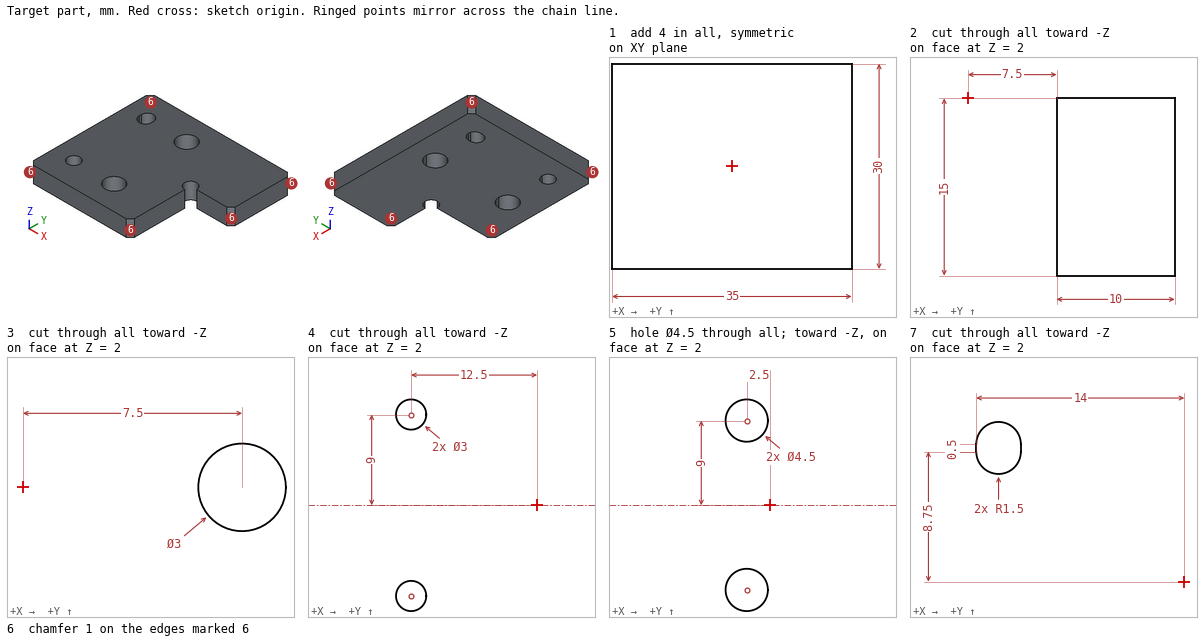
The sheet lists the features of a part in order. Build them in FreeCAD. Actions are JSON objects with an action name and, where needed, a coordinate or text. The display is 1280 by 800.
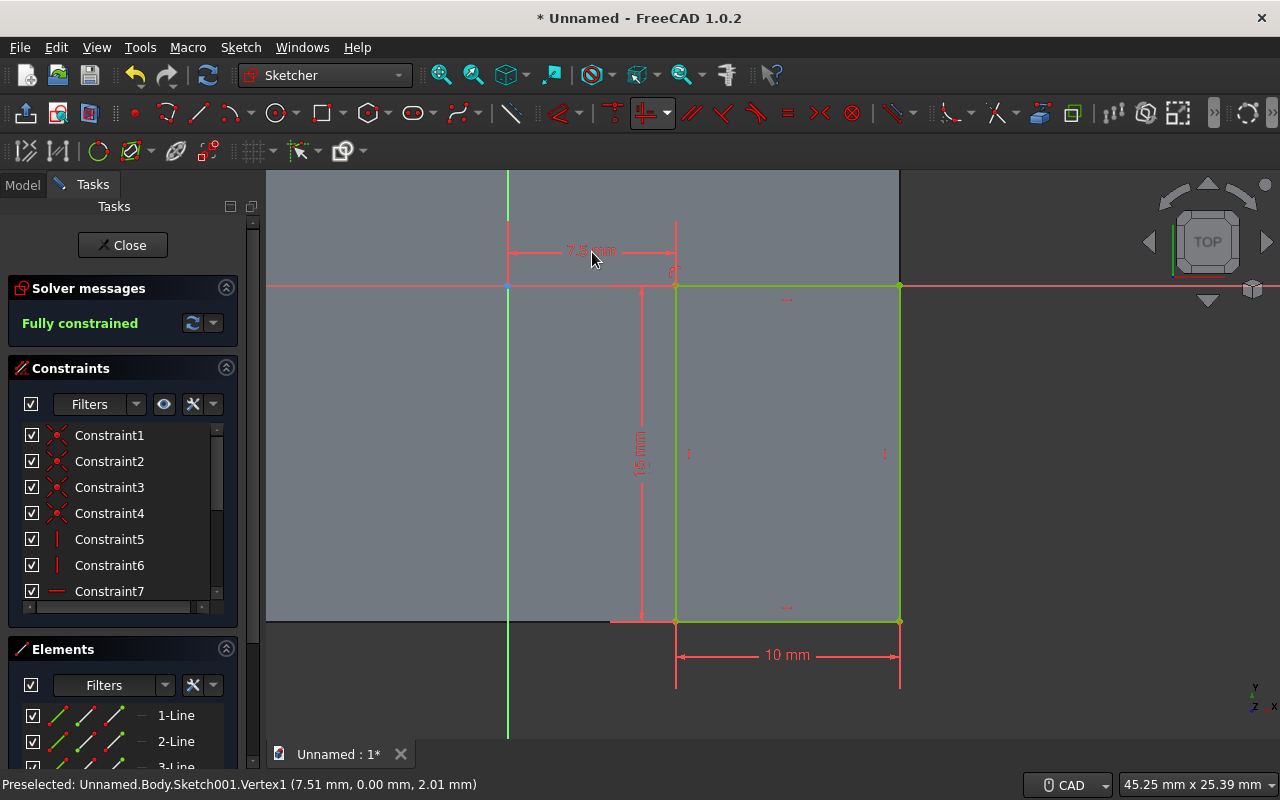
{"action": "left_click", "coordinate": [123, 245]}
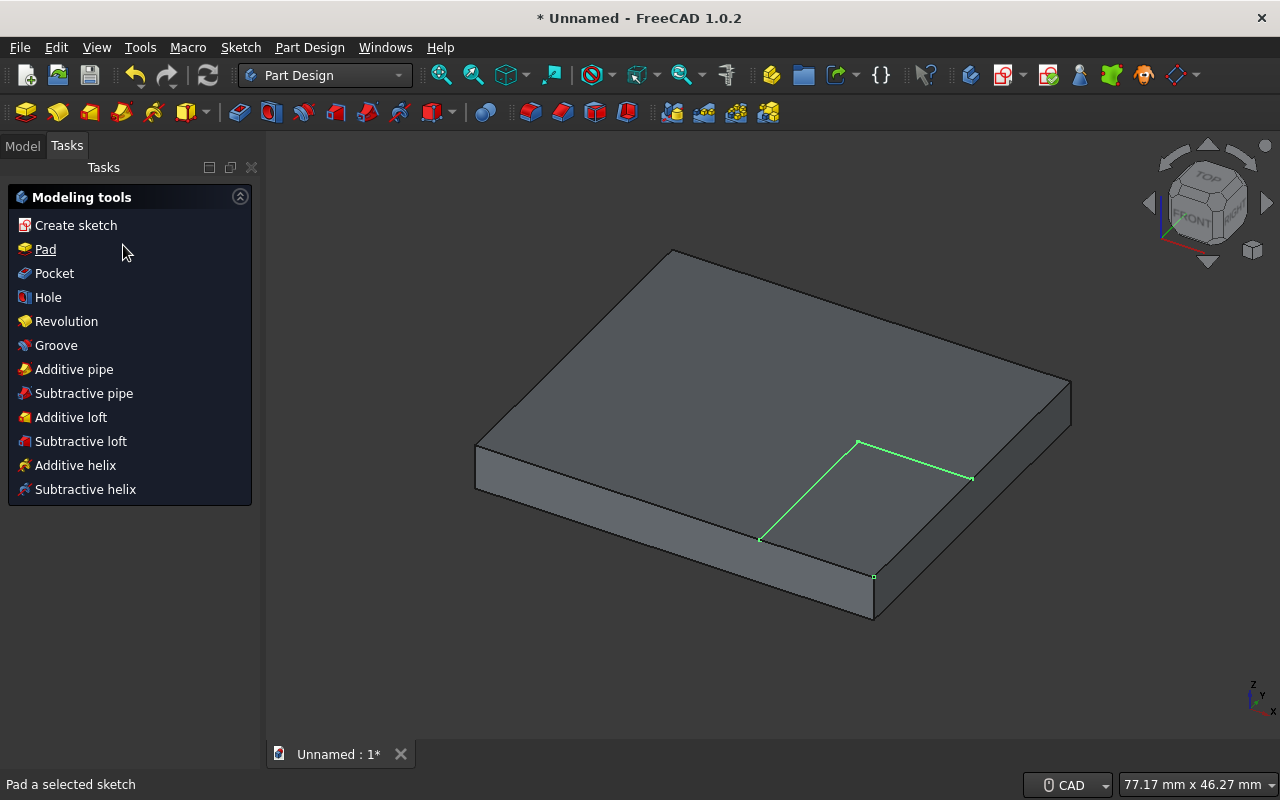
{"action": "left_click", "coordinate": [240, 112]}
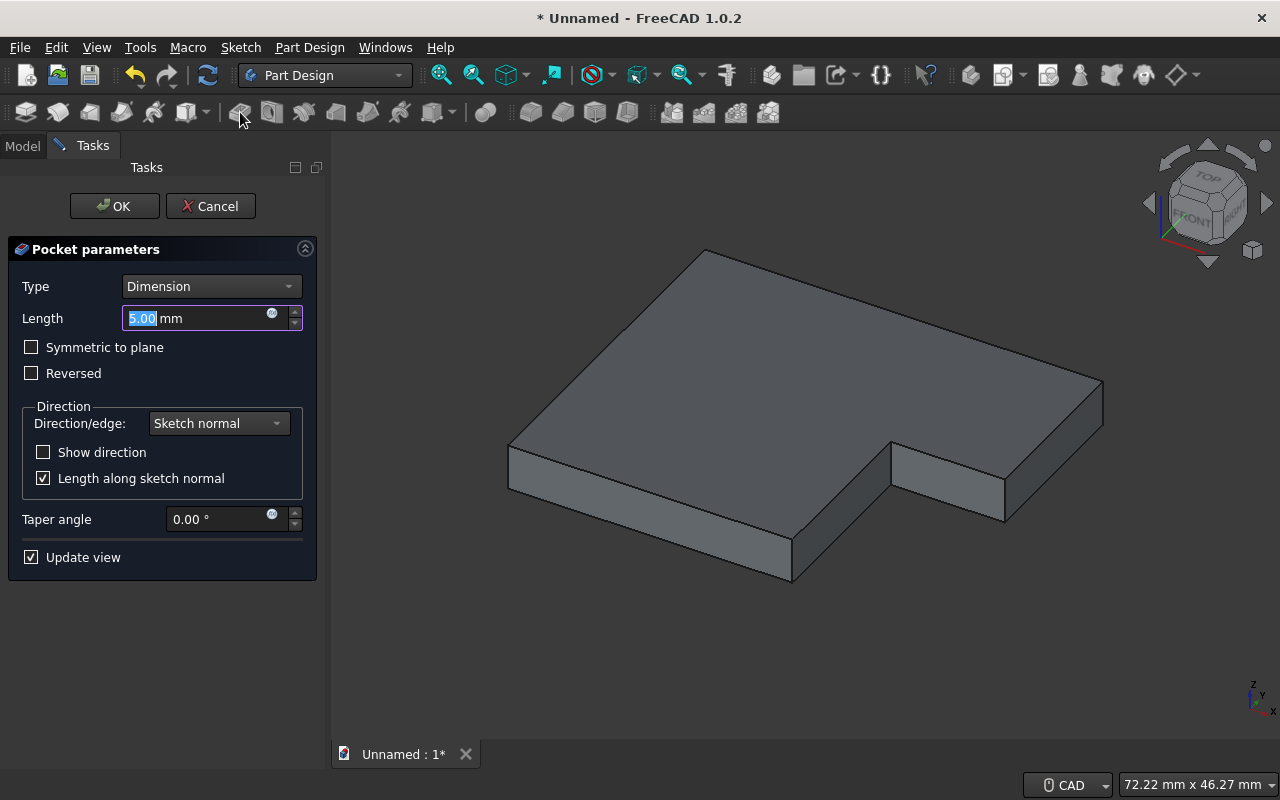
{"action": "left_click", "coordinate": [212, 286]}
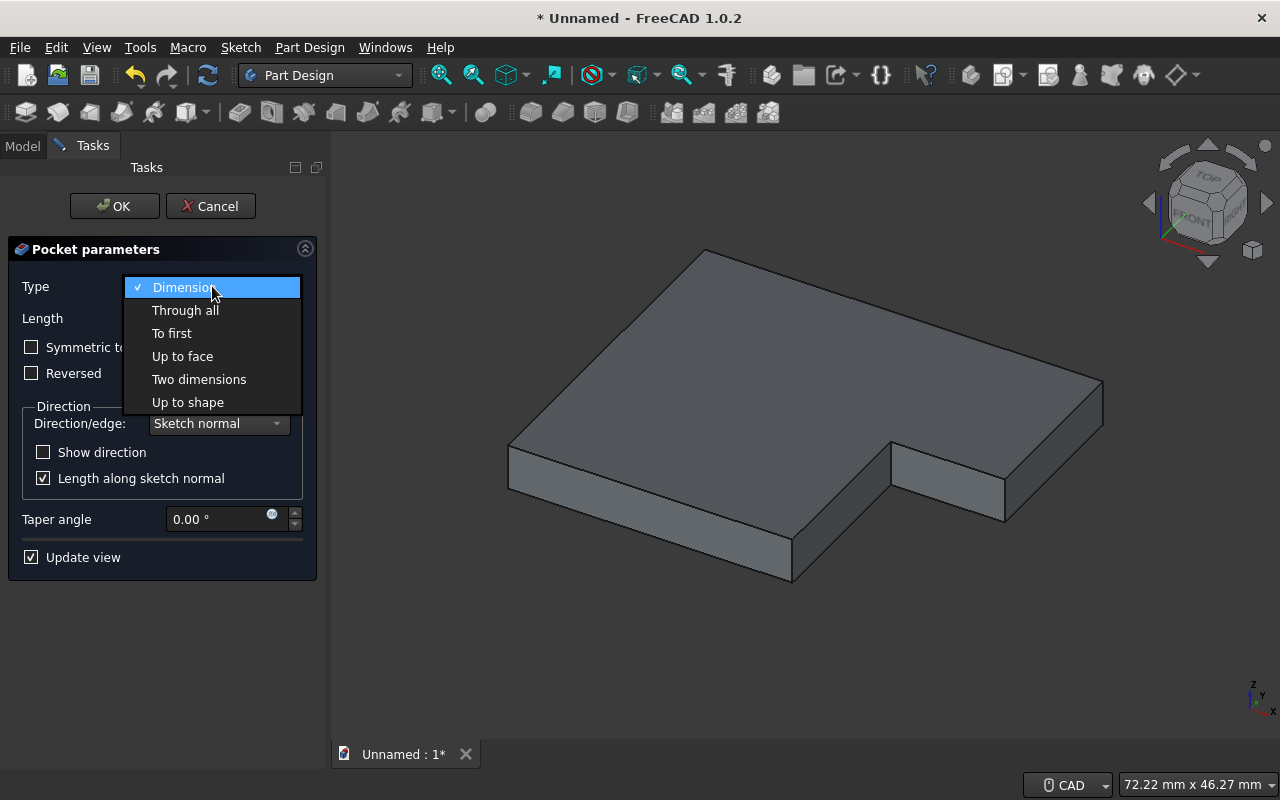
{"action": "left_click", "coordinate": [212, 310]}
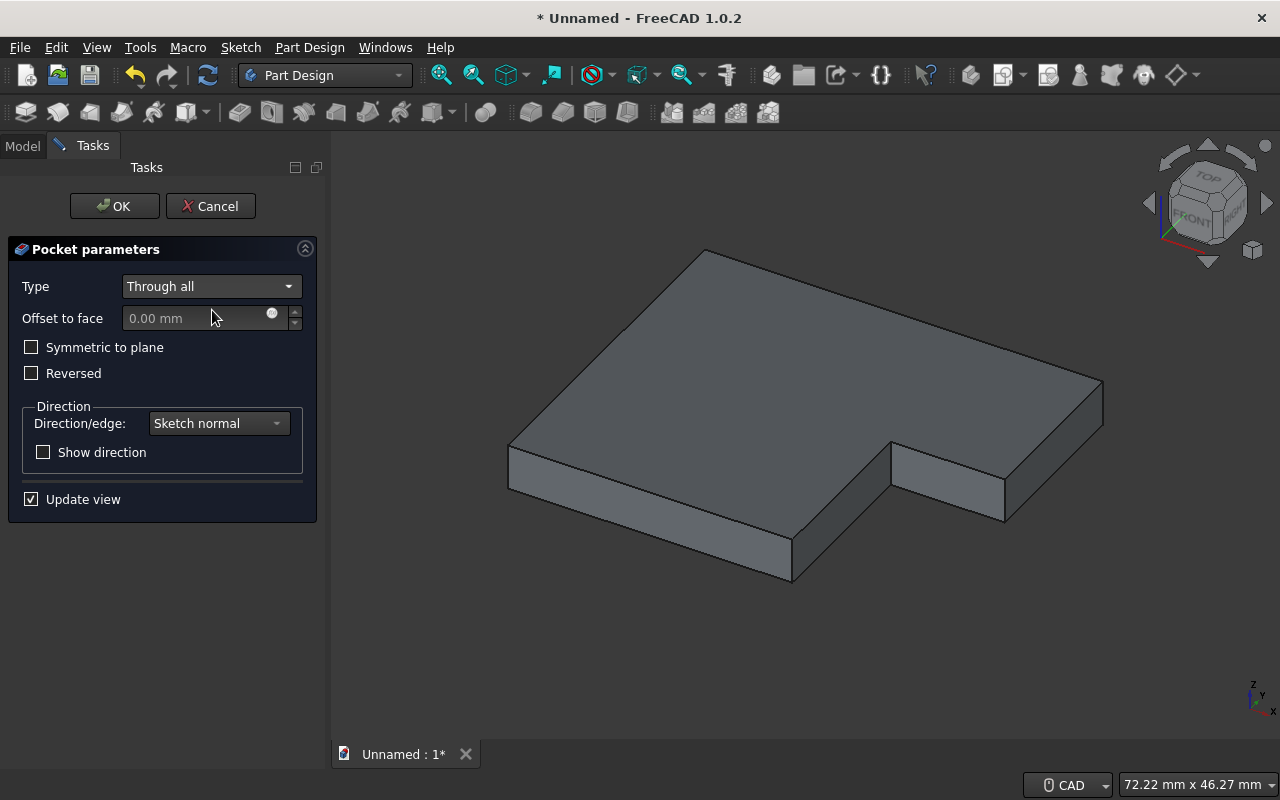
{"action": "left_click", "coordinate": [115, 206]}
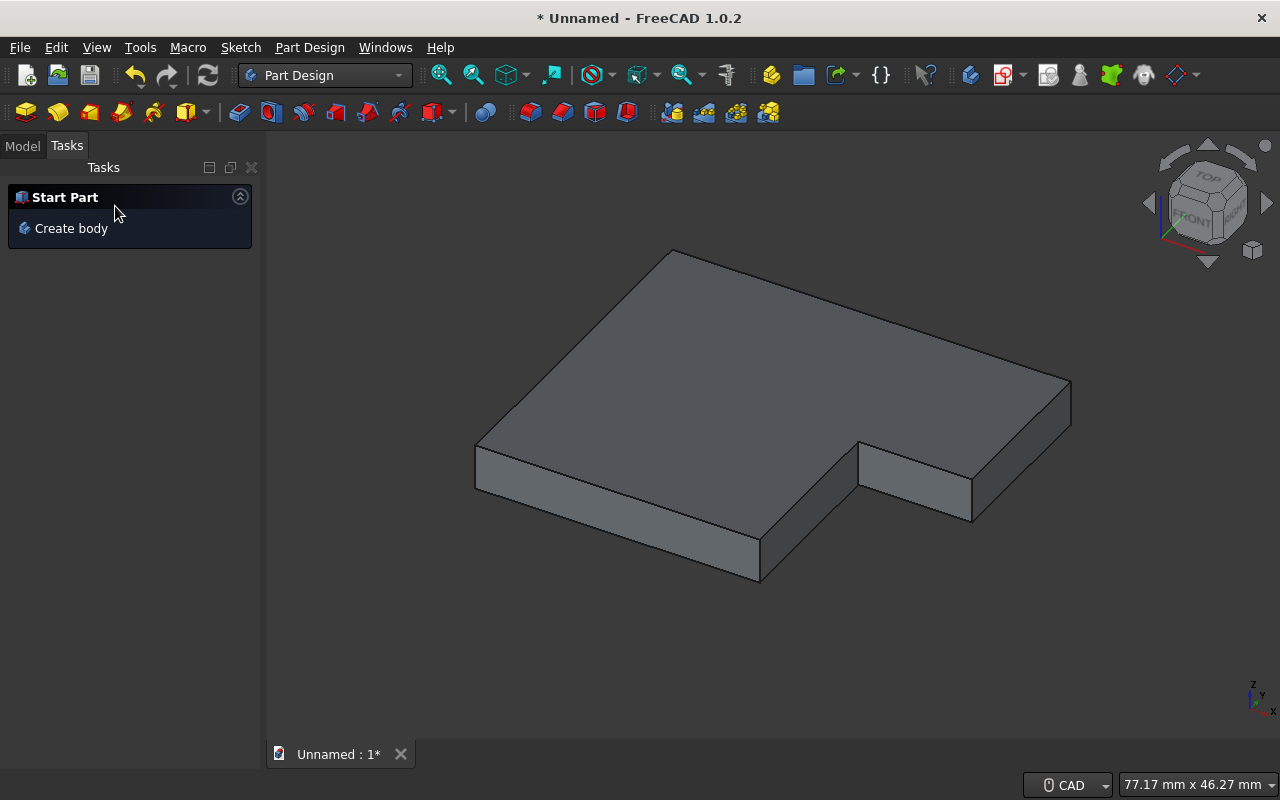
{"action": "left_click", "coordinate": [716, 394]}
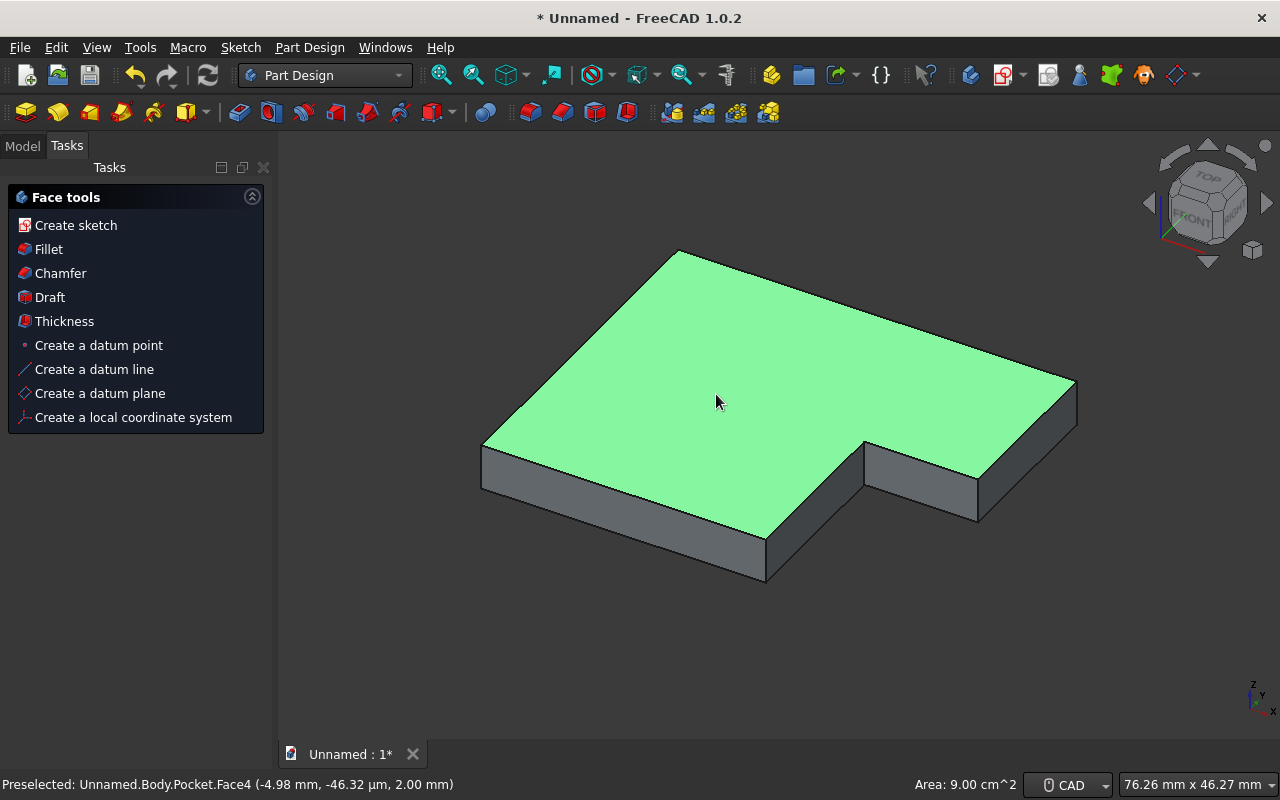
{"action": "left_click", "coordinate": [1004, 76]}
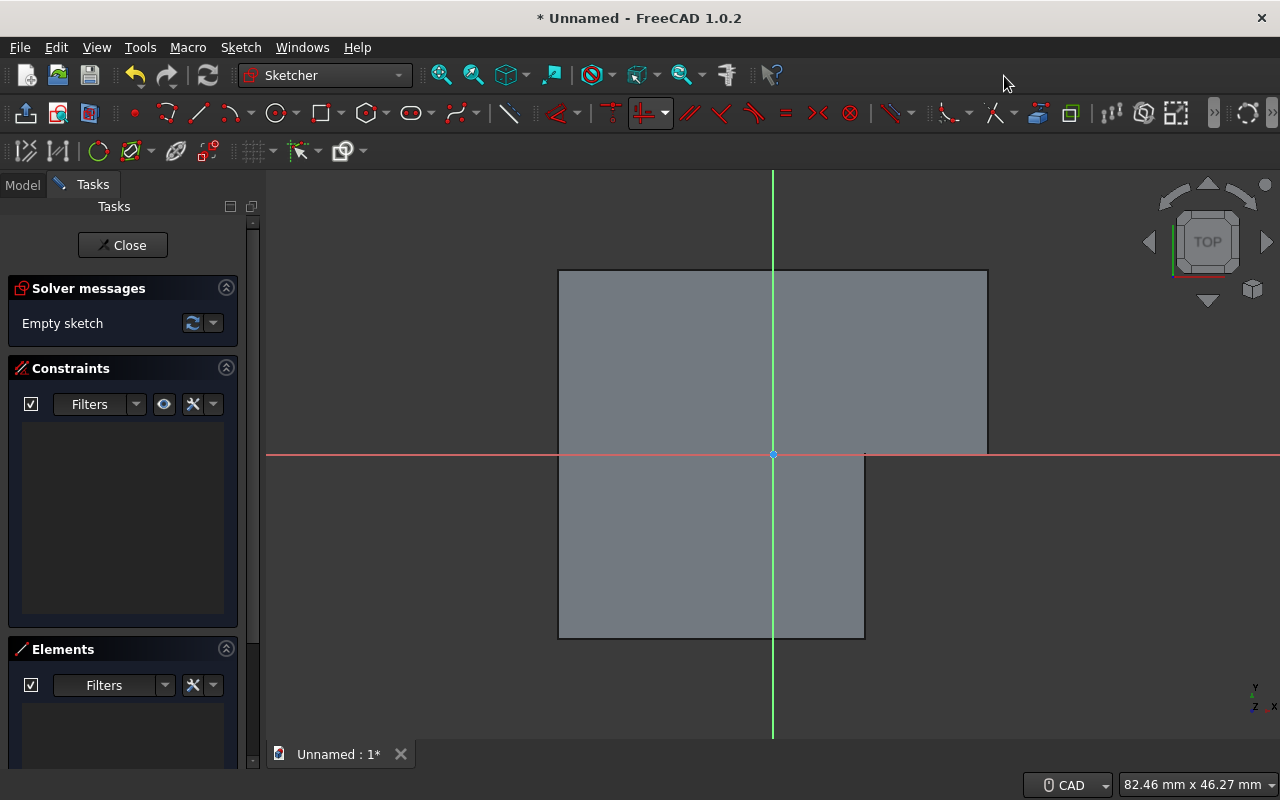
{"action": "scroll", "coordinate": [885, 454], "scroll_direction": "up", "scroll_amount": 11}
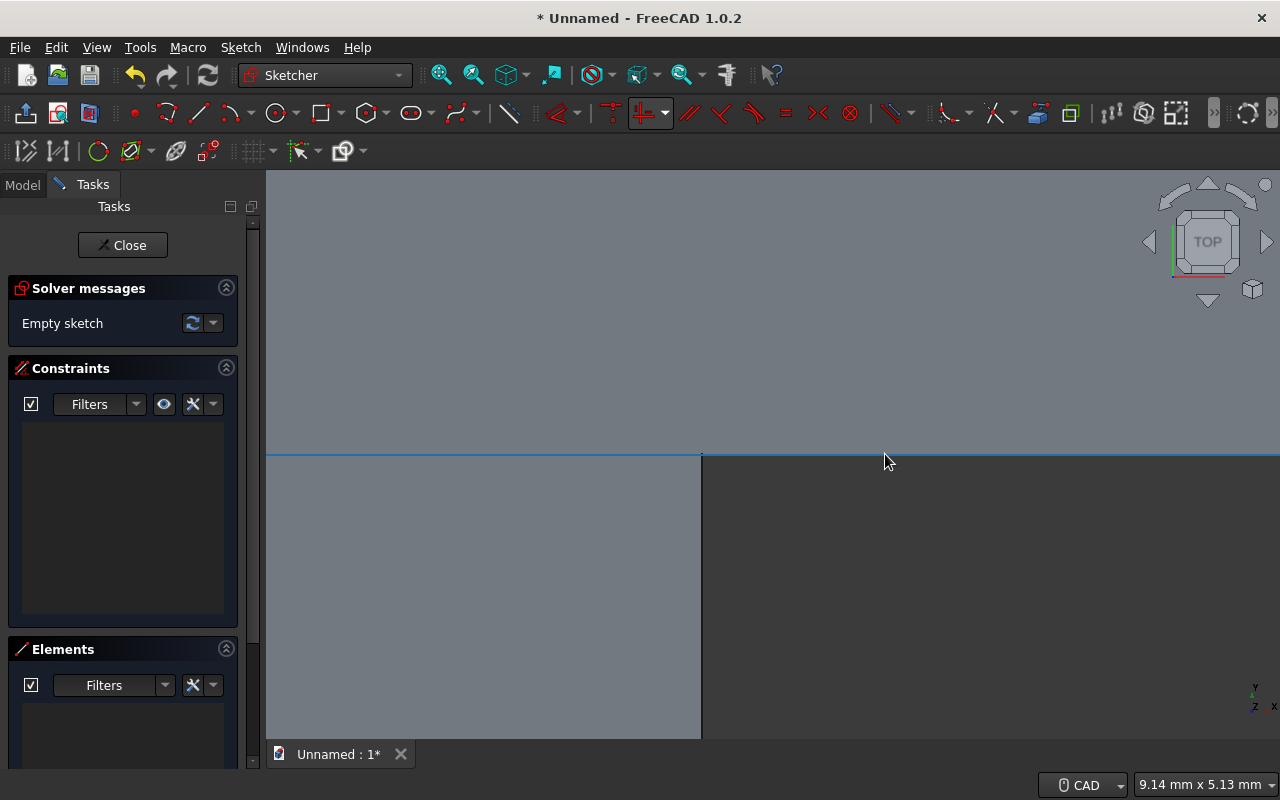
{"action": "key", "text": "g c"}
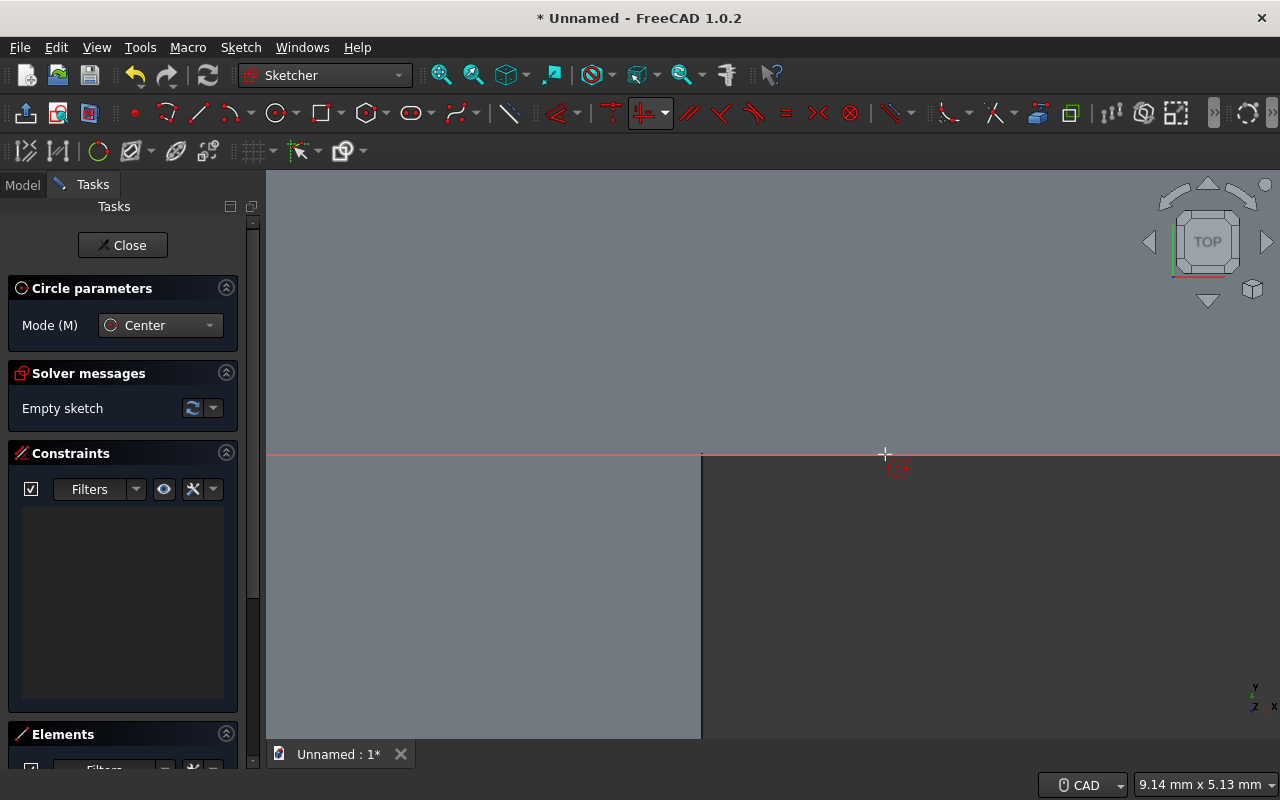
{"action": "left_click", "coordinate": [702, 454]}
{"action": "left_click", "coordinate": [819, 337]}
{"action": "key", "text": "Escape"}